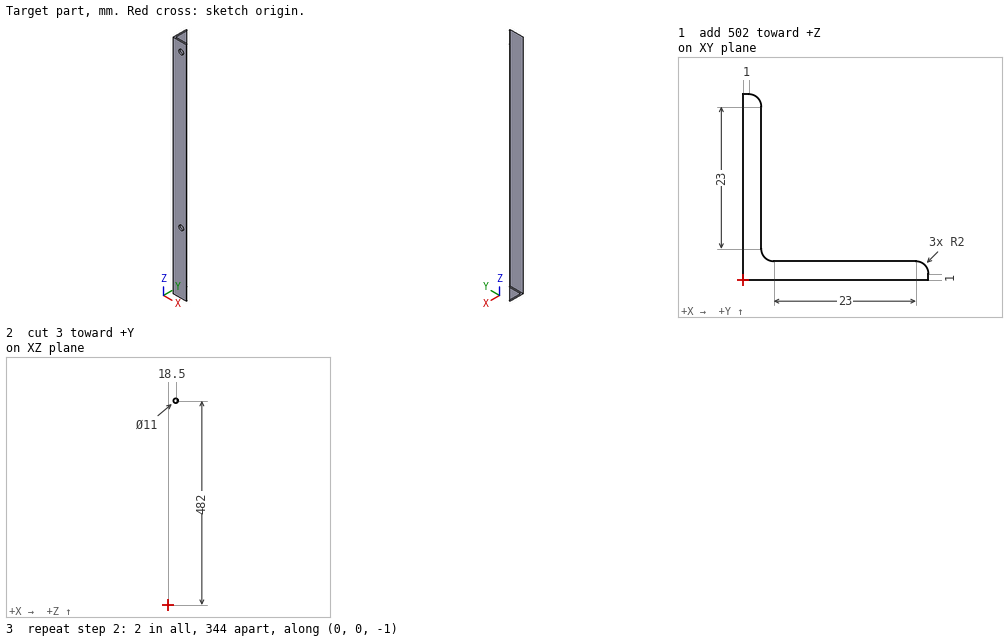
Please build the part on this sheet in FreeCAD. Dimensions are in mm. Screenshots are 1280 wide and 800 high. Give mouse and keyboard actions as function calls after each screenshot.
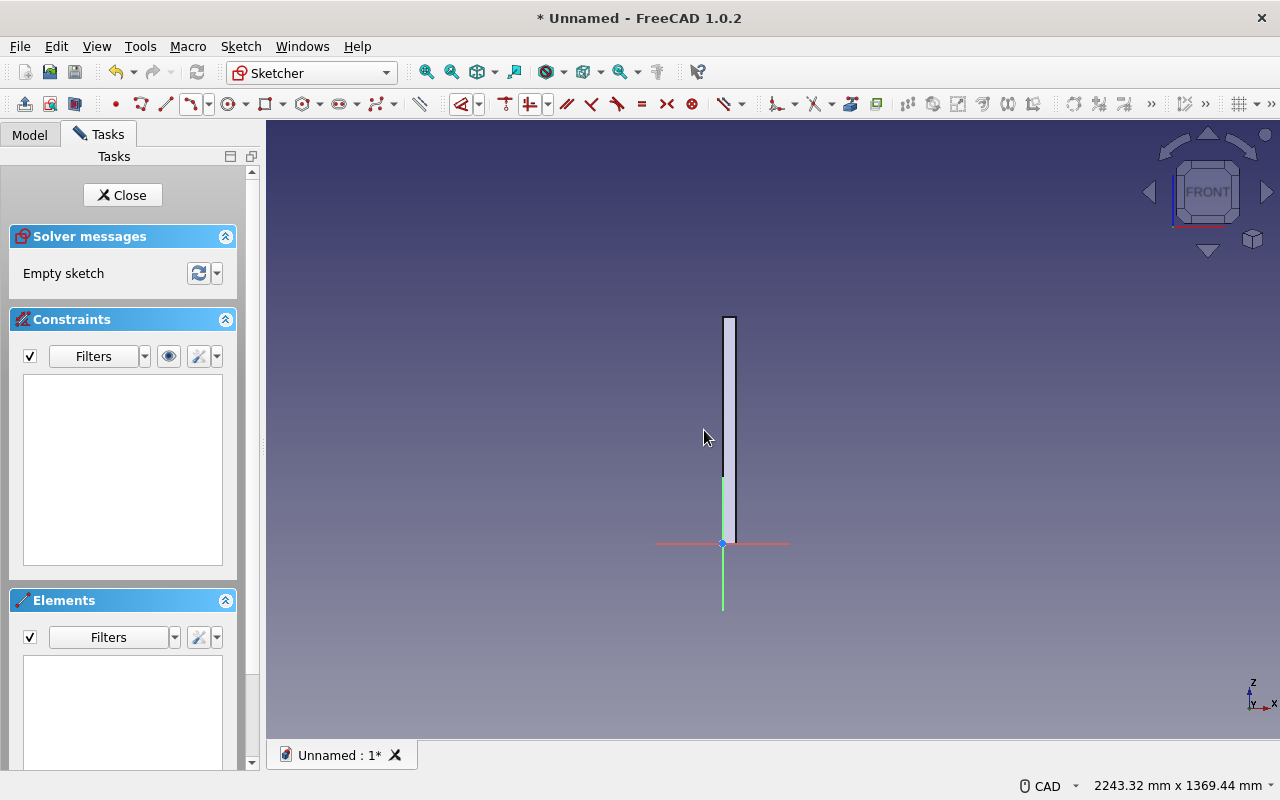
scroll(733, 320, up, 15)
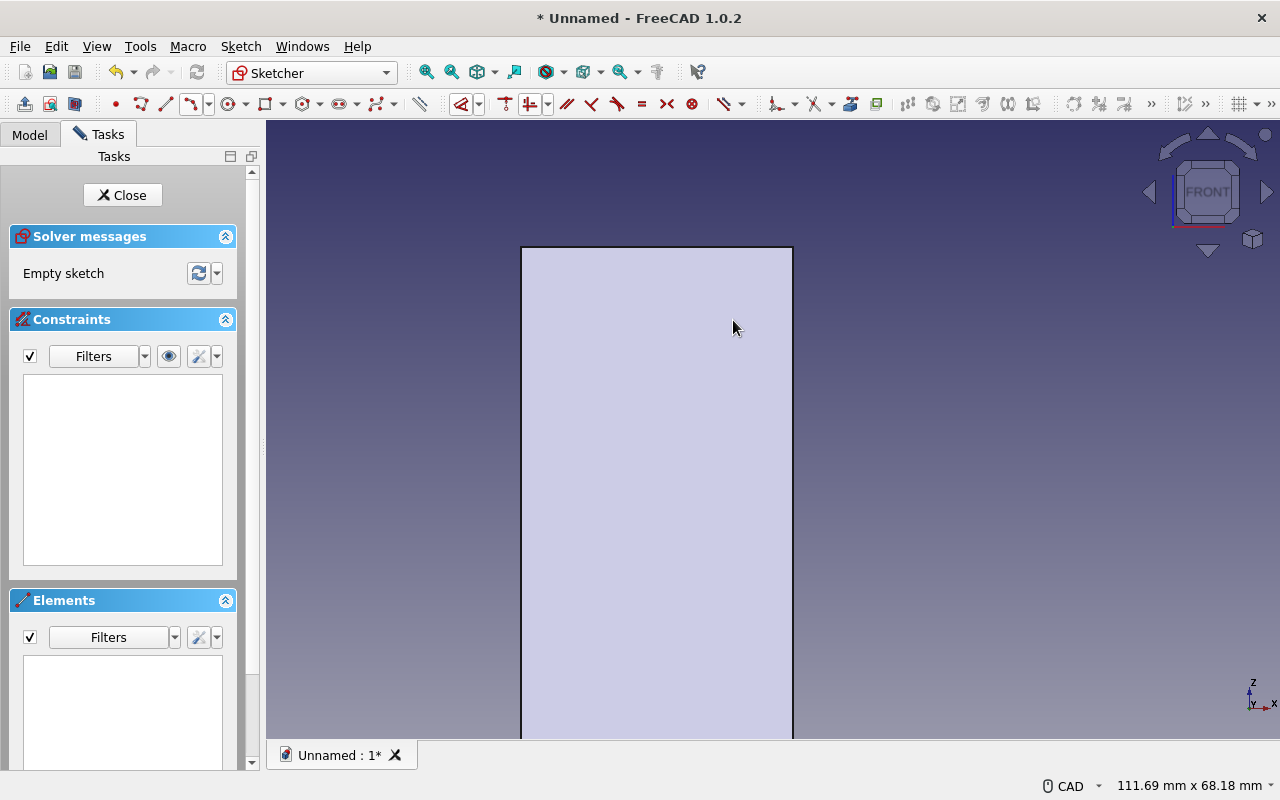
scroll(684, 428, up, 7)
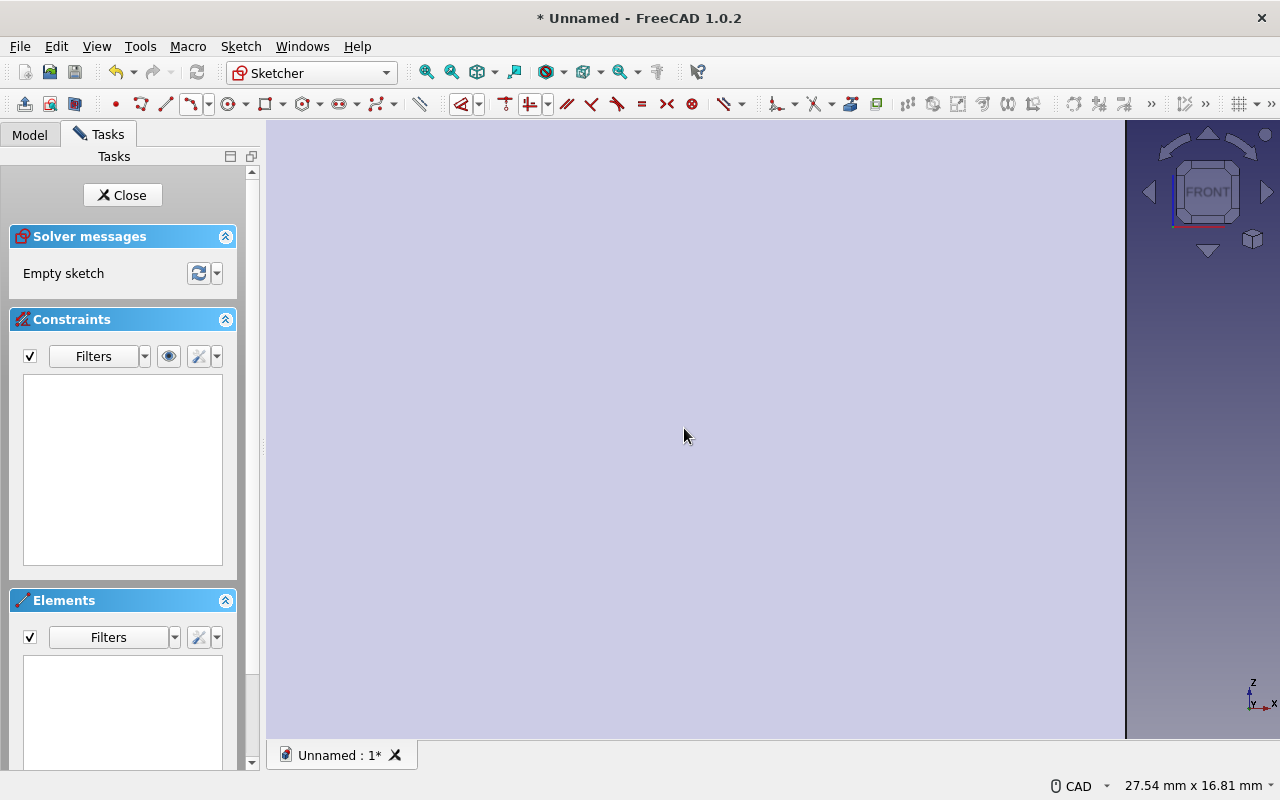
click(228, 104)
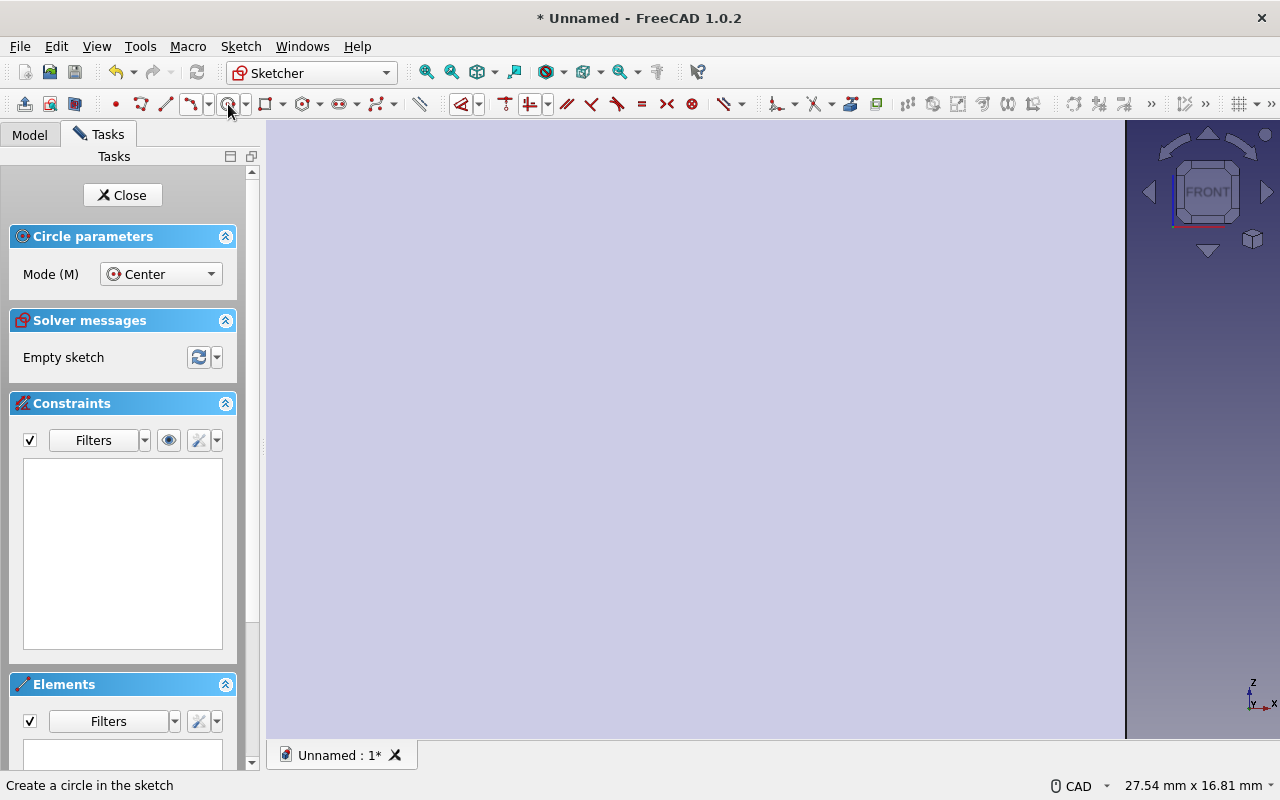
click(702, 429)
move(846, 286)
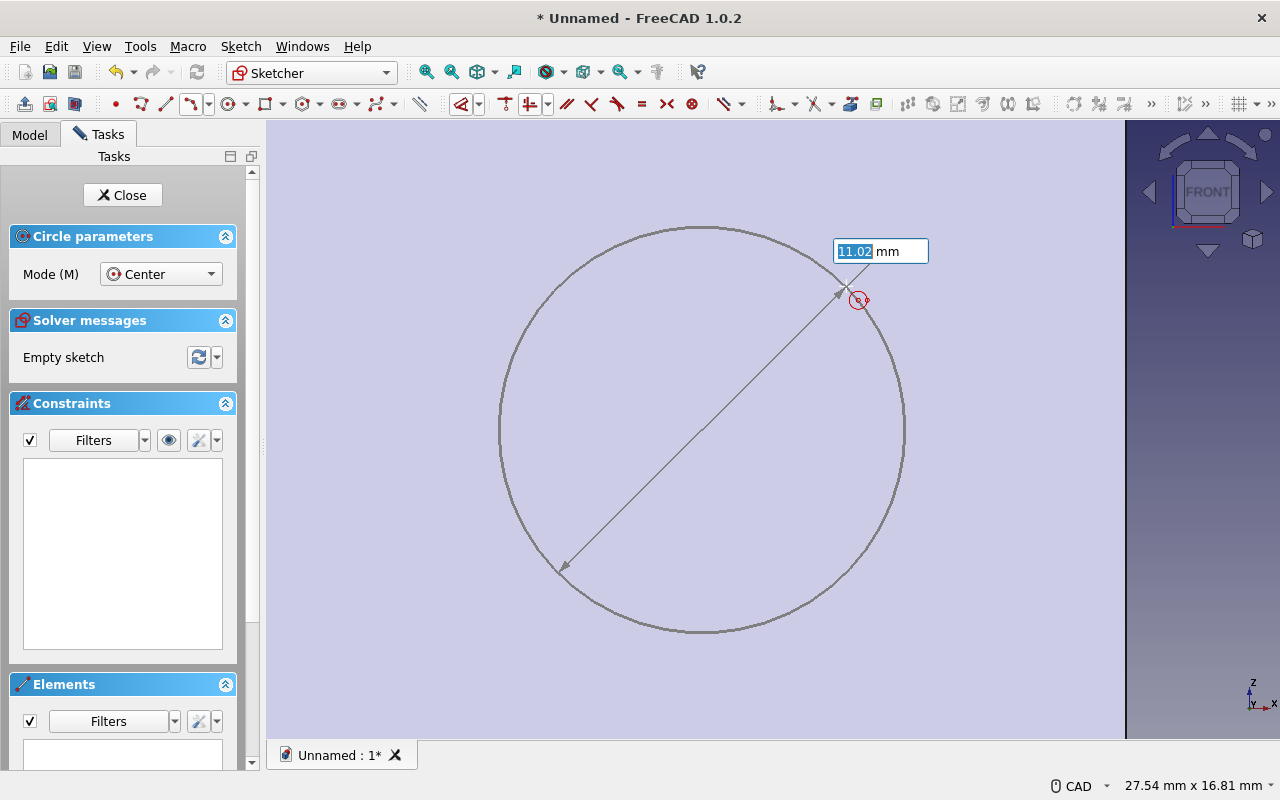
text(11)
key(Return)
key(Escape)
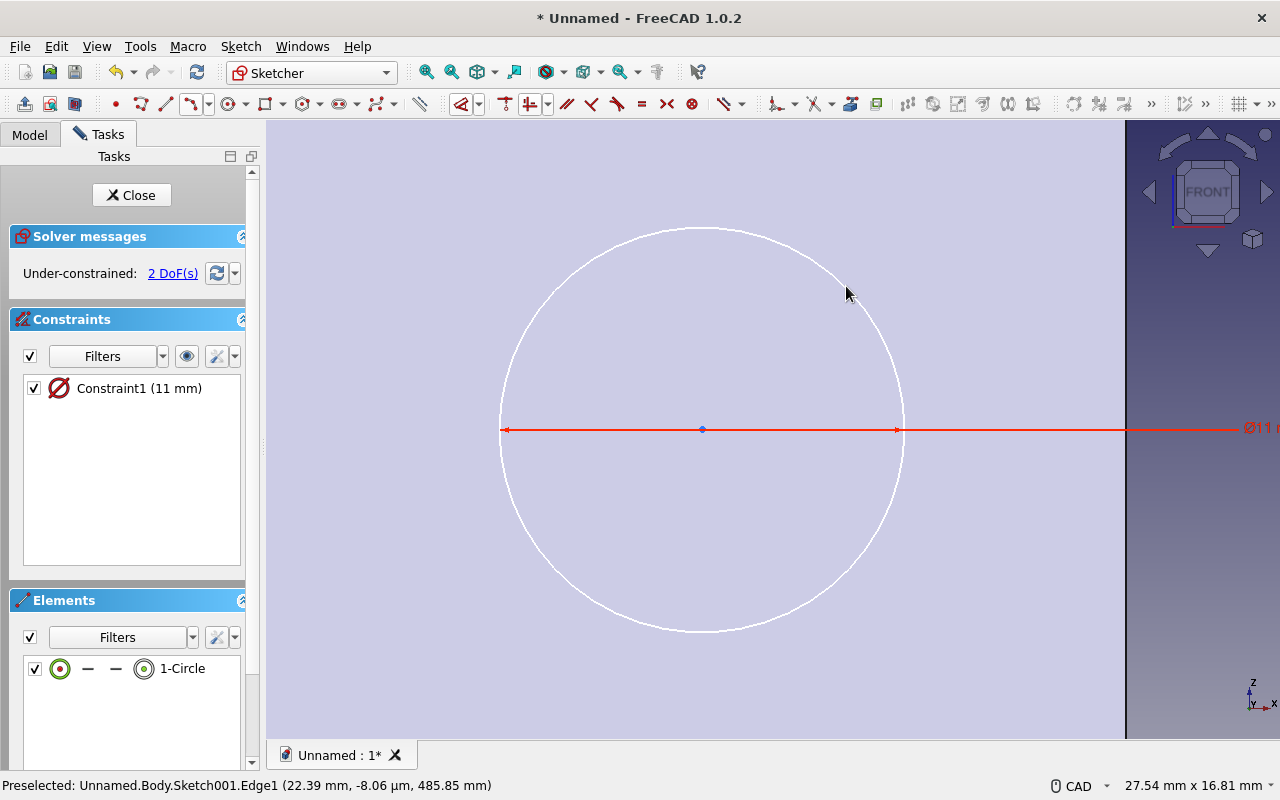
click(702, 430)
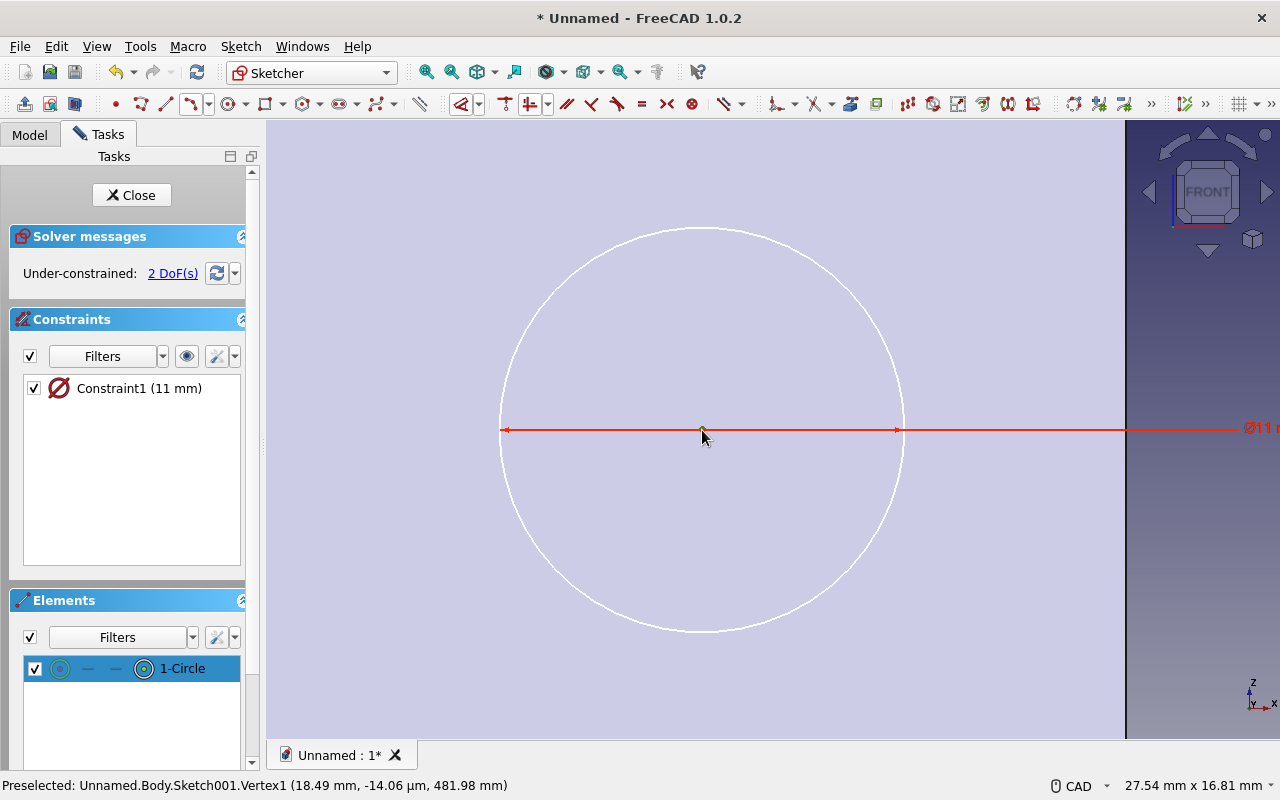
key(i)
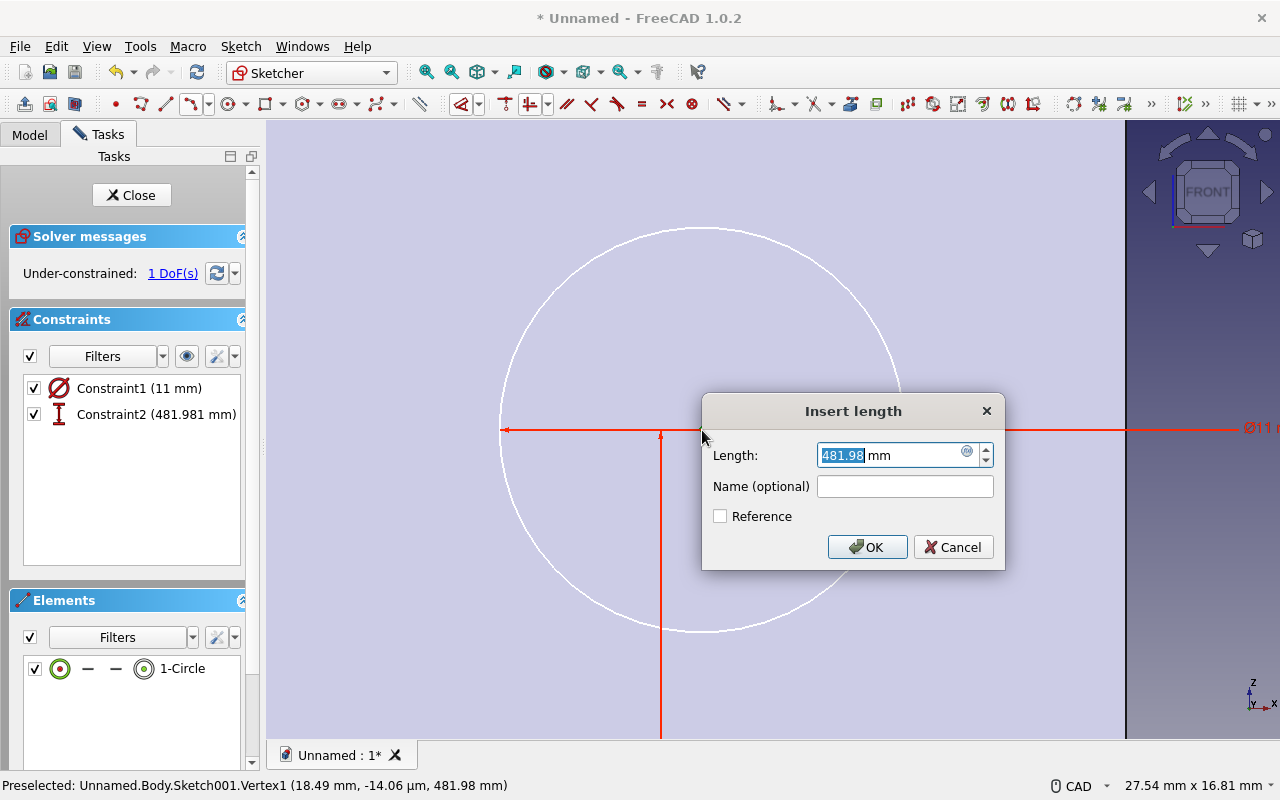
text(482)
key(Return)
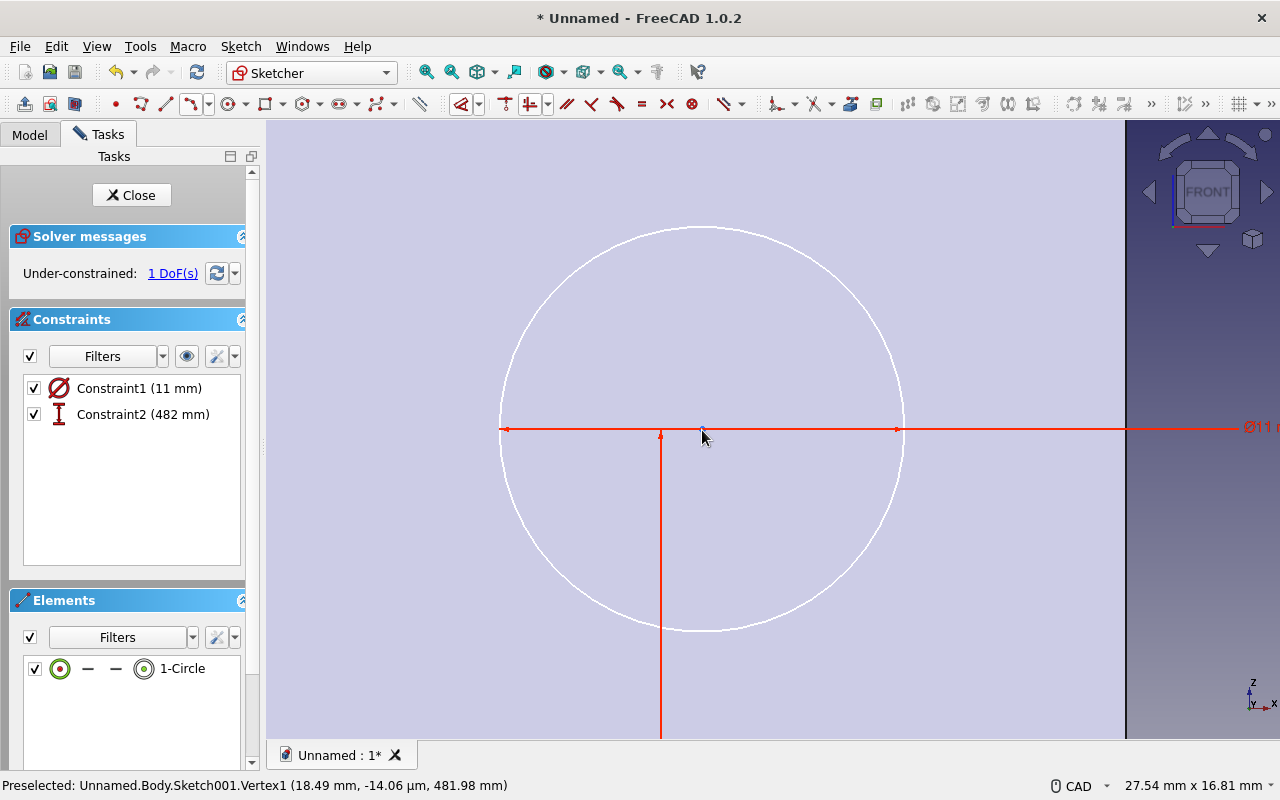
click(702, 429)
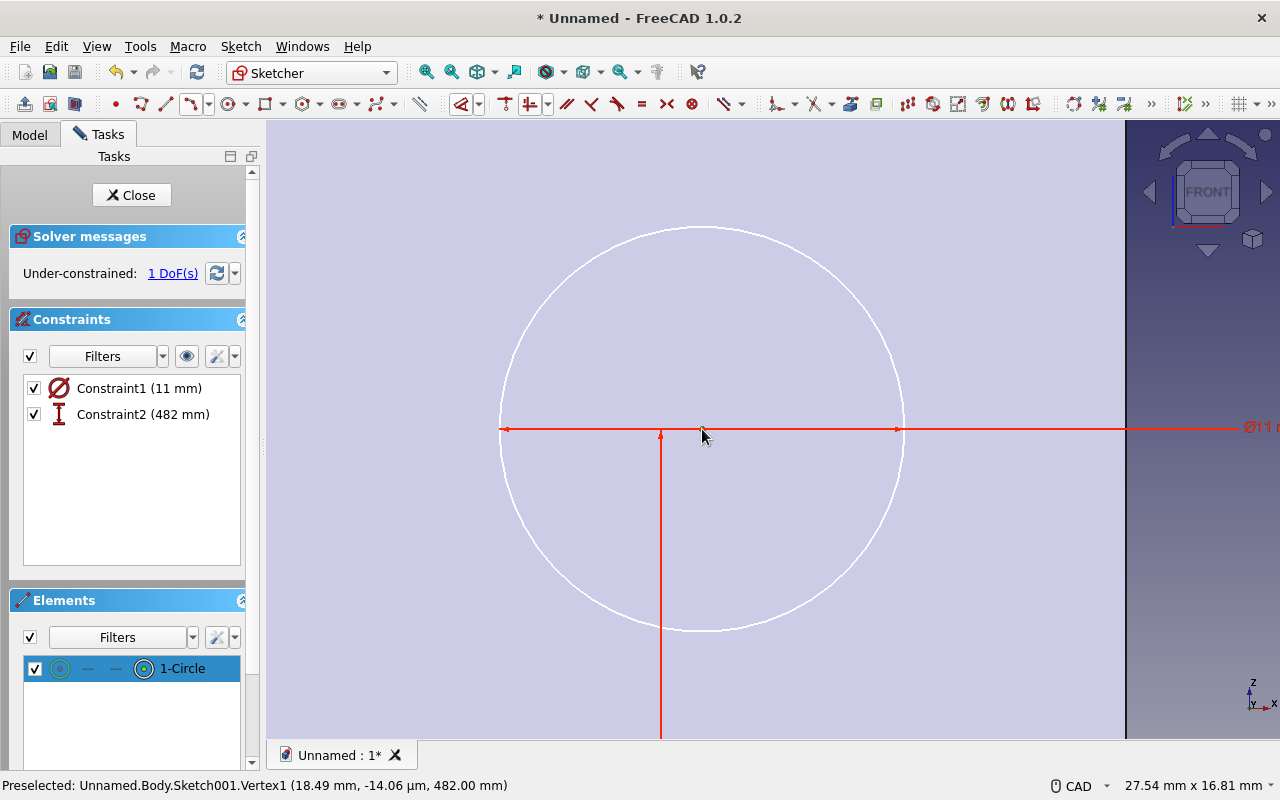
click(478, 104)